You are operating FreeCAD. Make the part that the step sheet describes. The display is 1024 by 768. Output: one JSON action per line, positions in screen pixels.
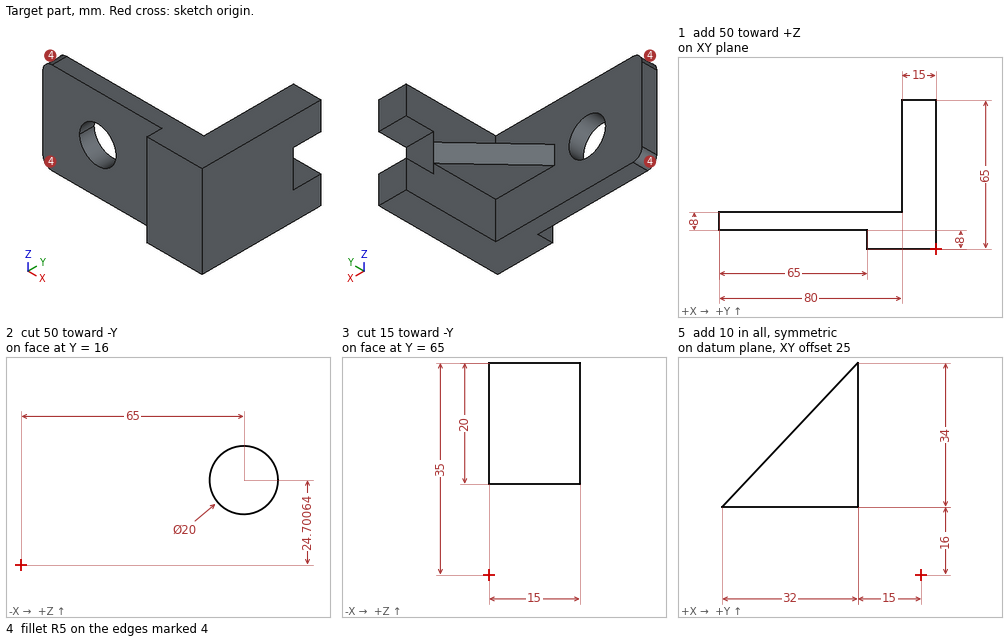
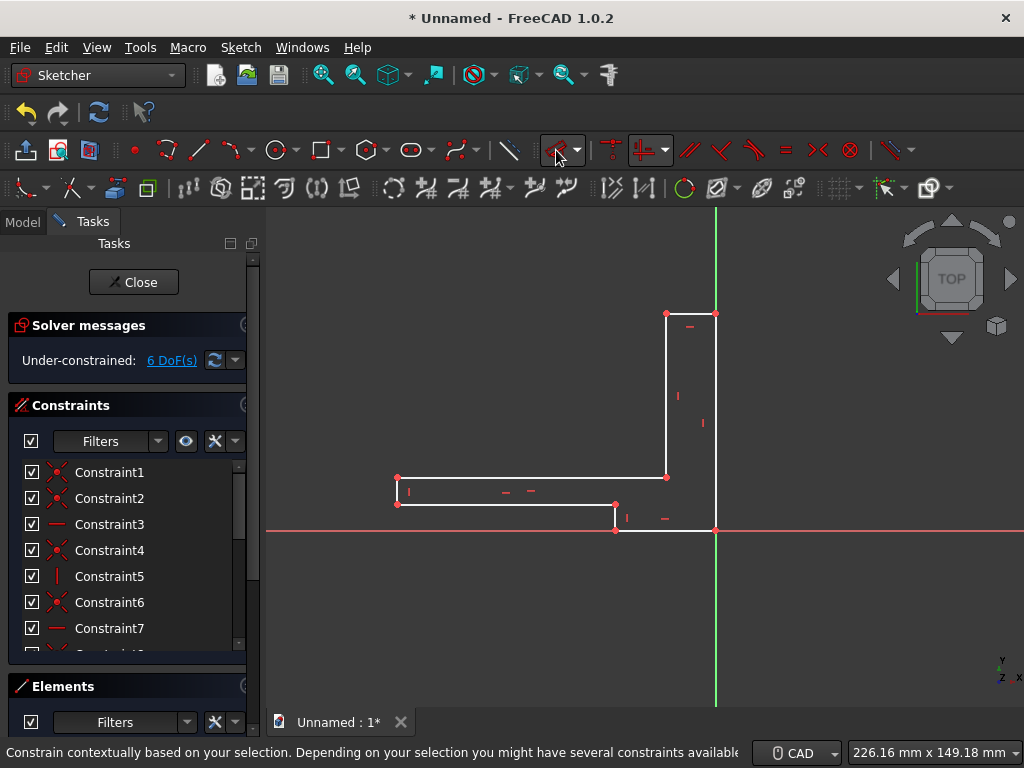
{"action": "scroll", "coordinate": [397, 489], "scroll_direction": "up", "scroll_amount": 2}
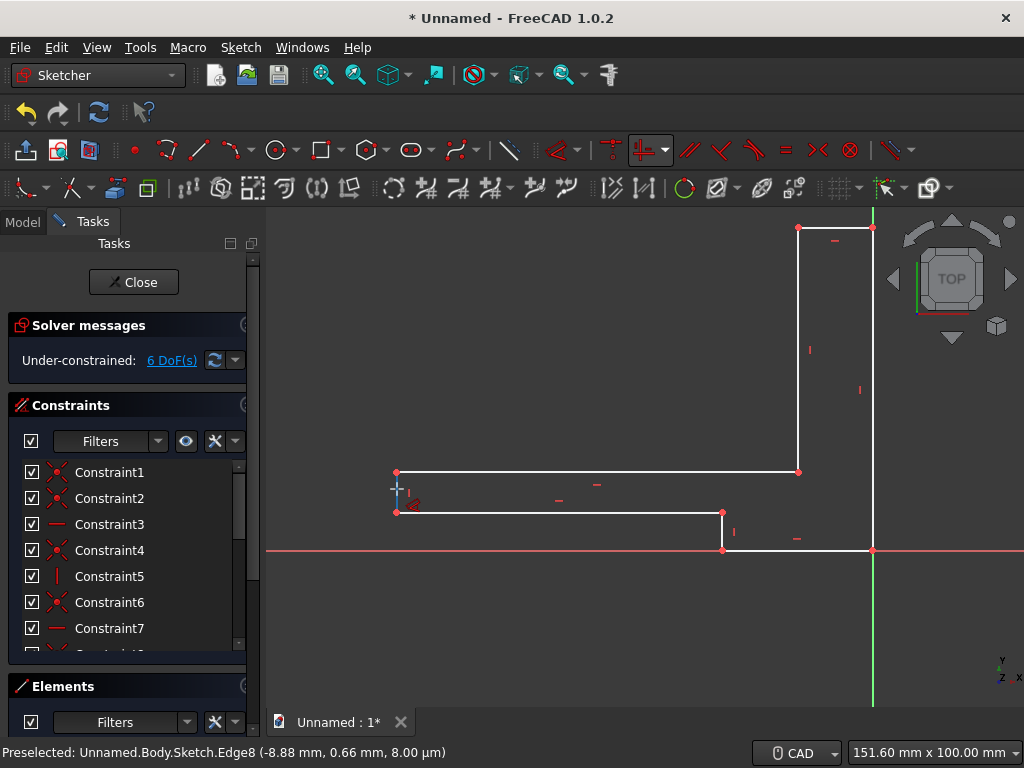
{"action": "left_click", "coordinate": [397, 488]}
{"action": "left_click", "coordinate": [363, 492]}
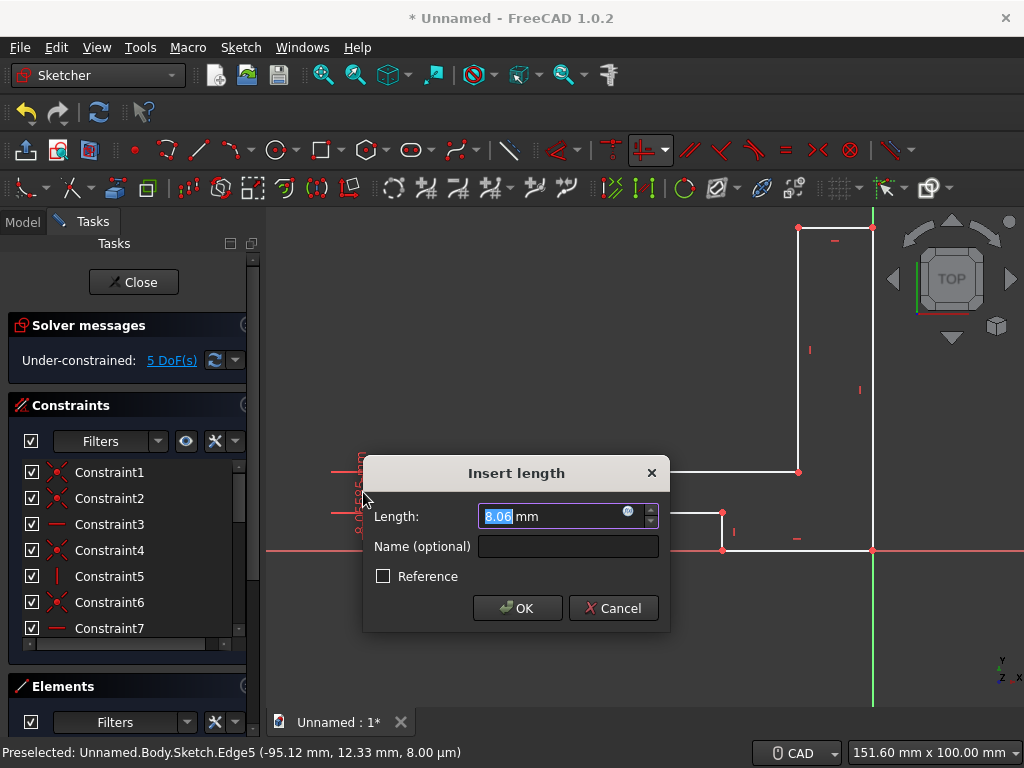
{"action": "type", "text": "8"}
{"action": "key", "text": "Return"}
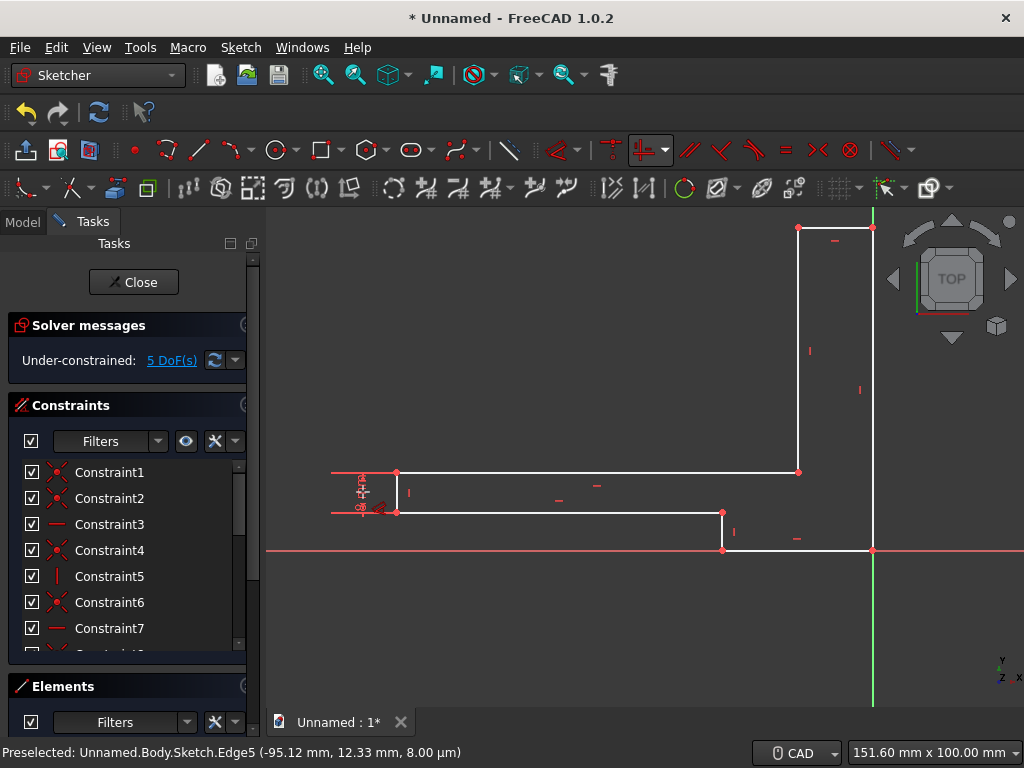
{"action": "left_click", "coordinate": [722, 524]}
{"action": "left_click", "coordinate": [756, 532]}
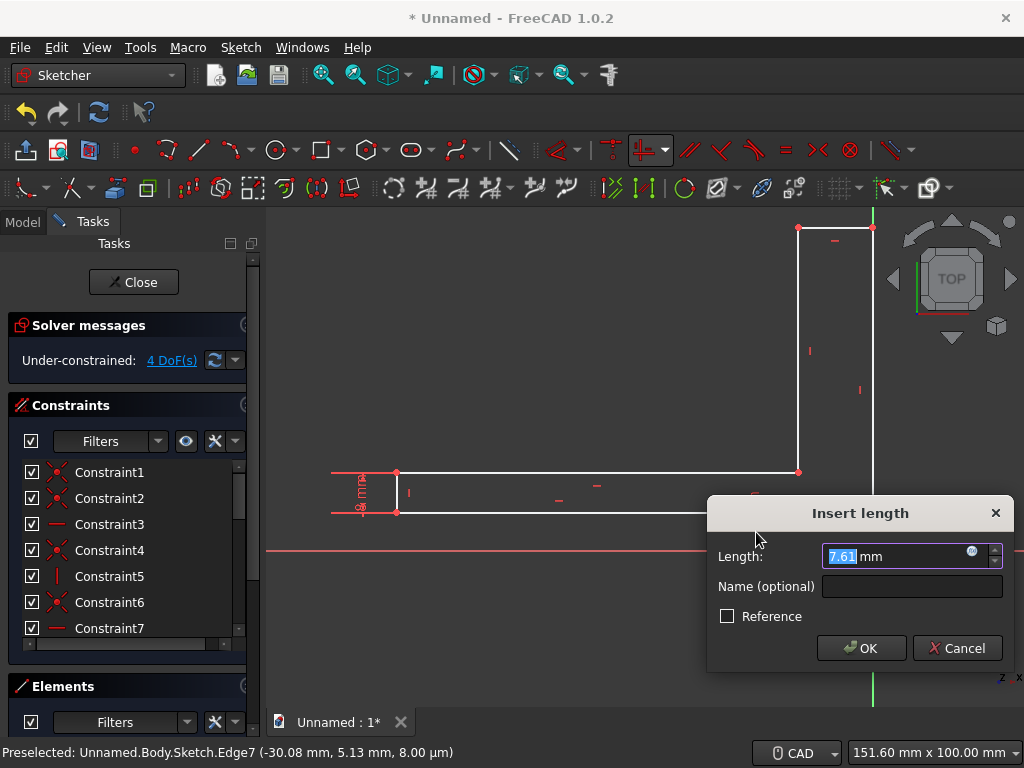
{"action": "type", "text": "8"}
{"action": "key", "text": "Return"}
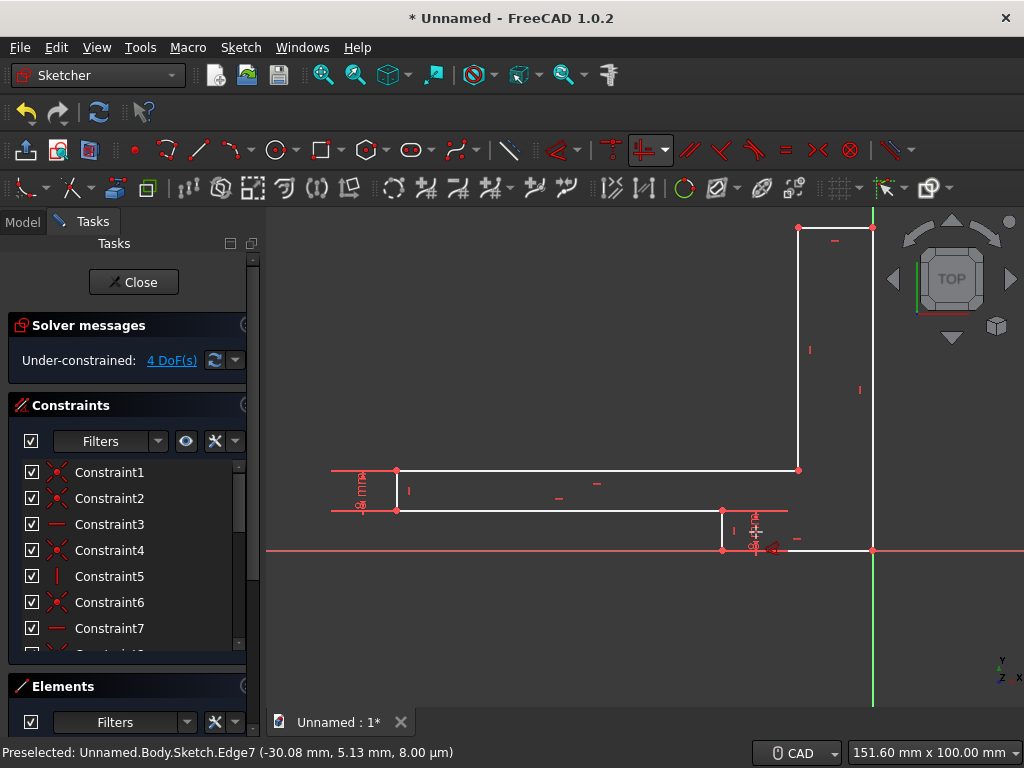
{"action": "scroll", "coordinate": [312, 679], "scroll_direction": "down", "scroll_amount": 1}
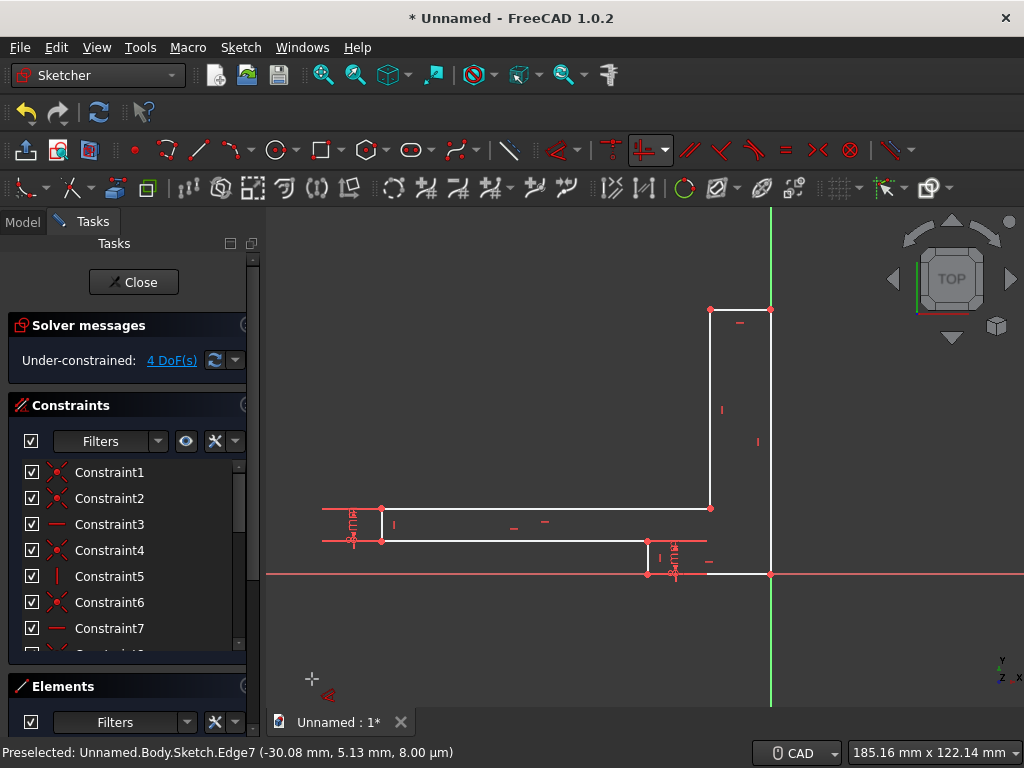
{"action": "left_click", "coordinate": [771, 495]}
{"action": "left_click", "coordinate": [805, 442]}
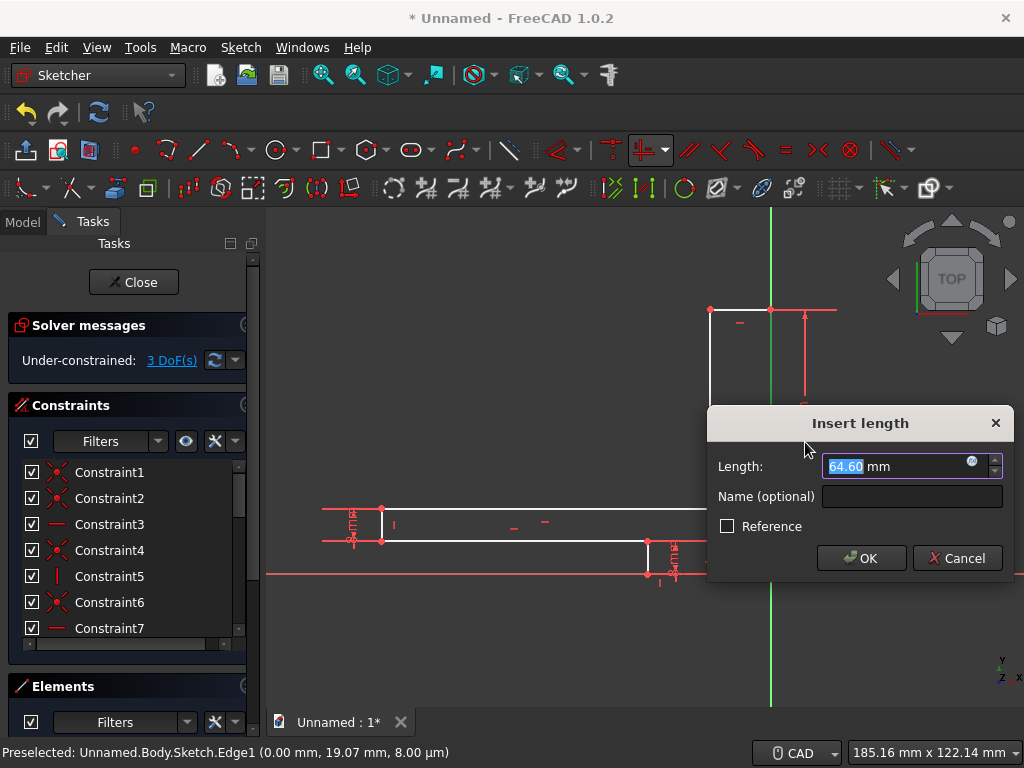
{"action": "type", "text": "65"}
{"action": "key", "text": "Return"}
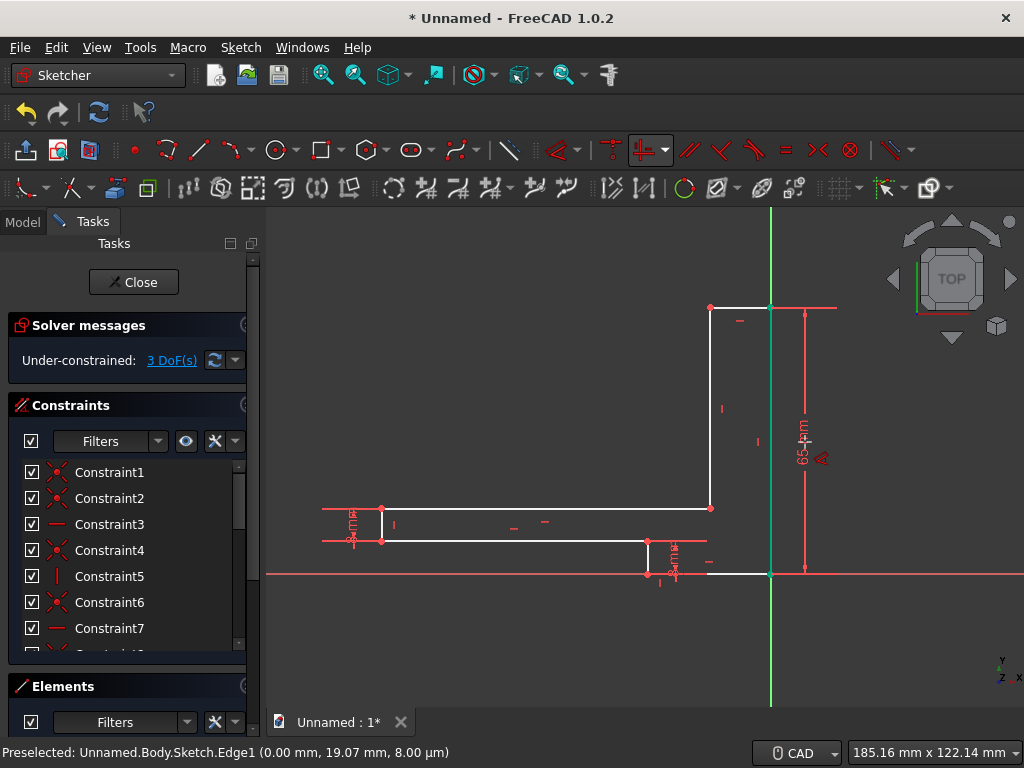
{"action": "left_click", "coordinate": [753, 308]}
{"action": "left_click", "coordinate": [741, 274]}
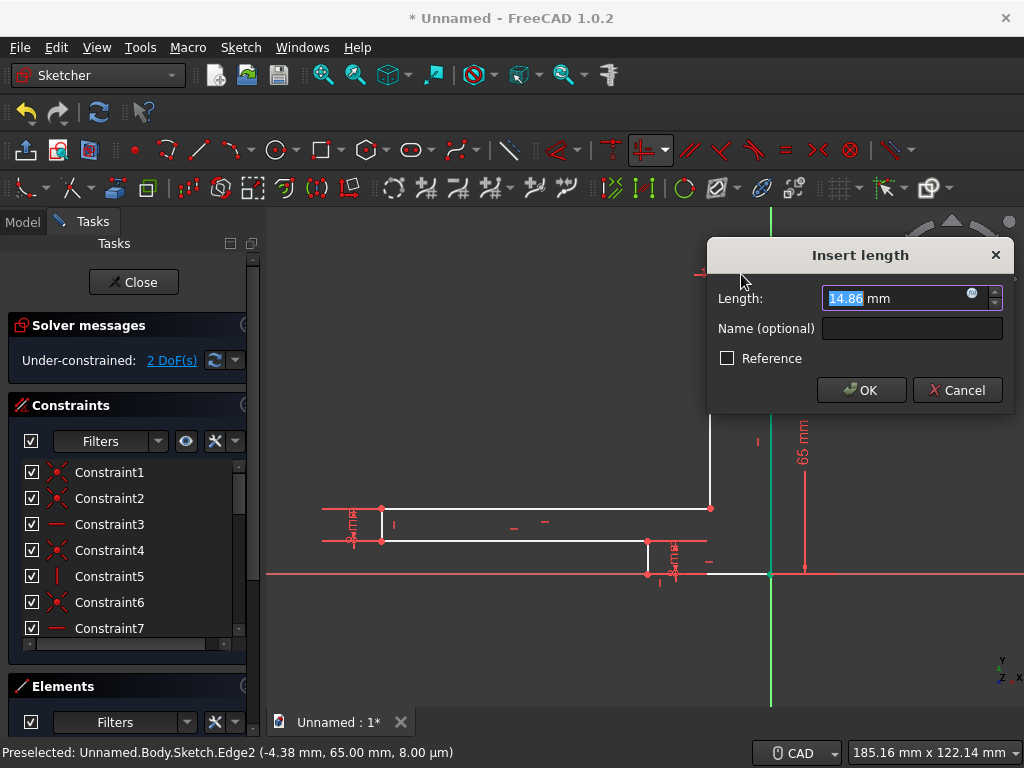
{"action": "type", "text": "15"}
{"action": "key", "text": "Return"}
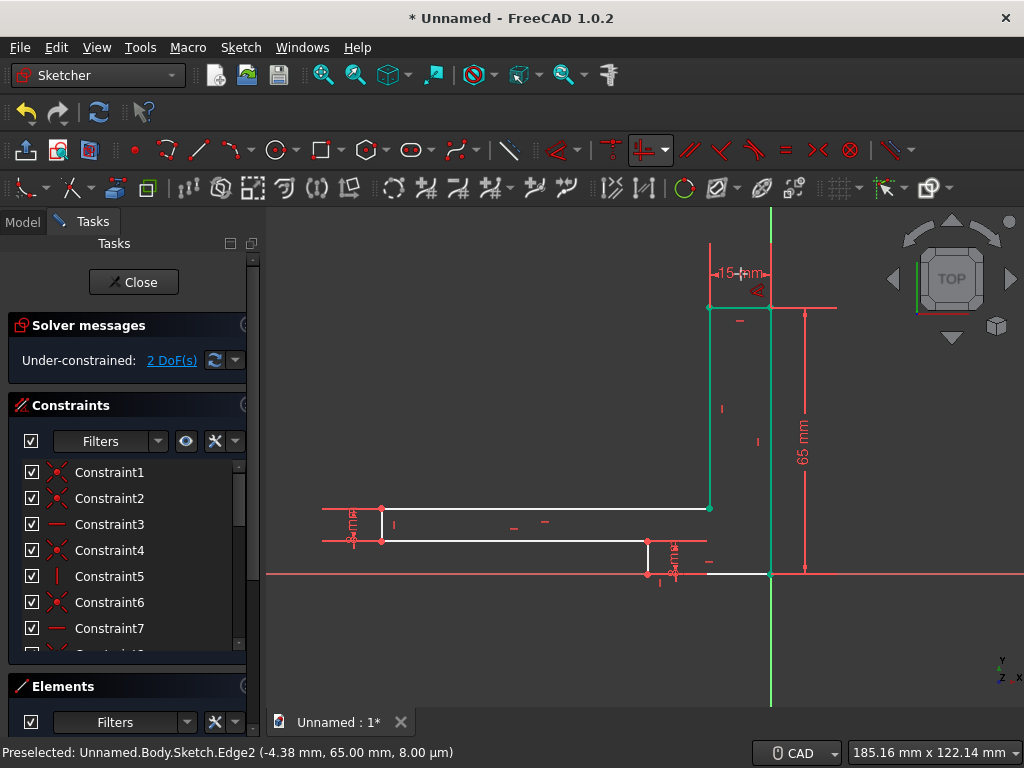
{"action": "left_click", "coordinate": [611, 509]}
{"action": "left_click", "coordinate": [546, 475]}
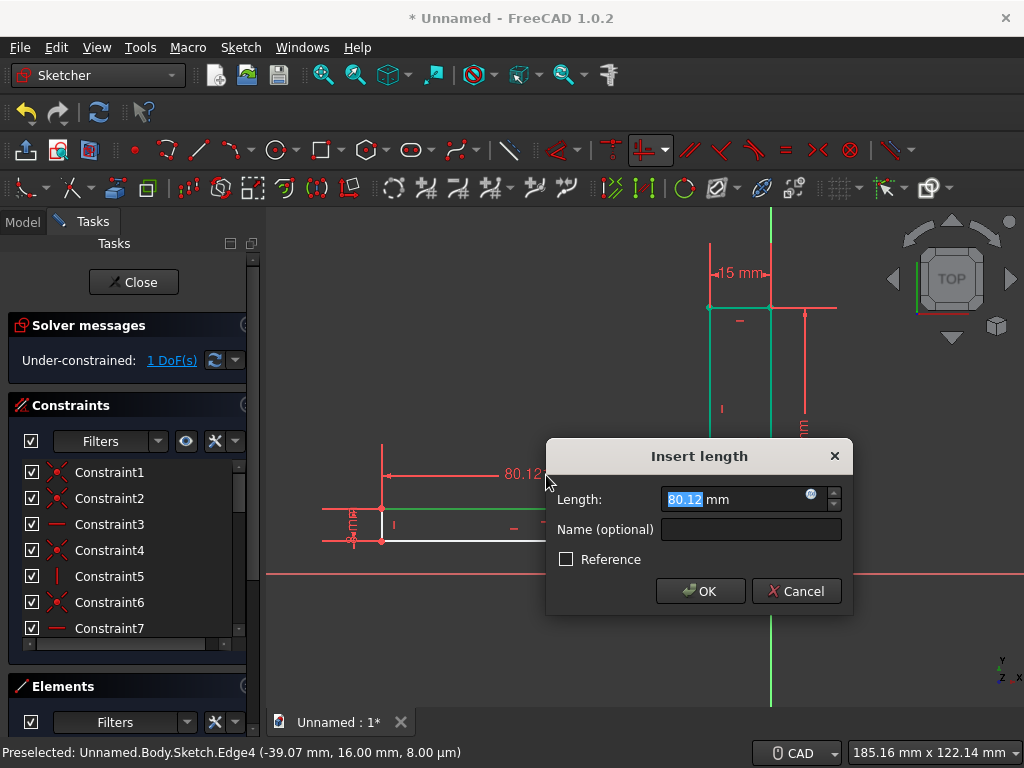
{"action": "type", "text": "80"}
{"action": "key", "text": "Return"}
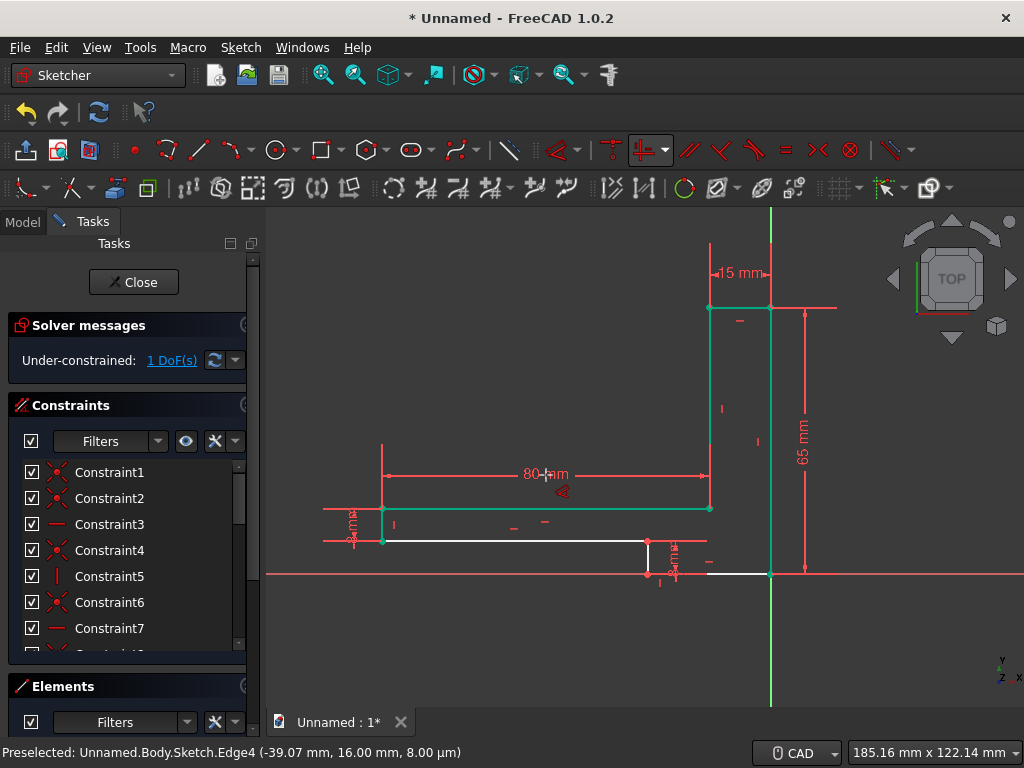
{"action": "left_click", "coordinate": [462, 541]}
{"action": "left_click", "coordinate": [515, 599]}